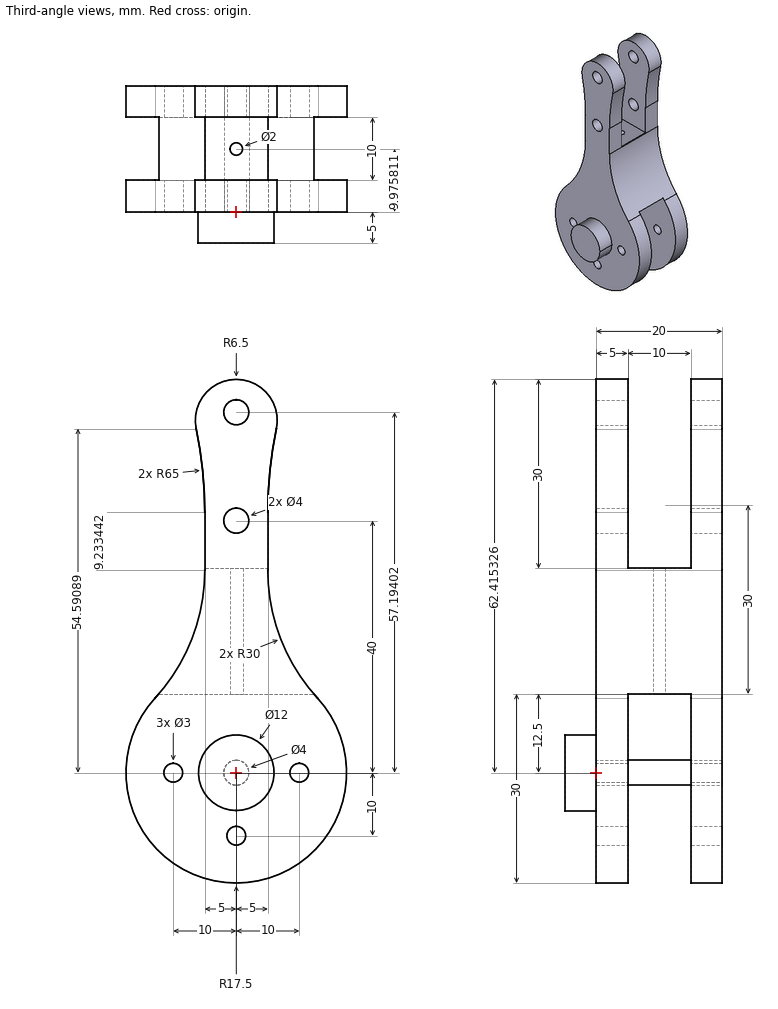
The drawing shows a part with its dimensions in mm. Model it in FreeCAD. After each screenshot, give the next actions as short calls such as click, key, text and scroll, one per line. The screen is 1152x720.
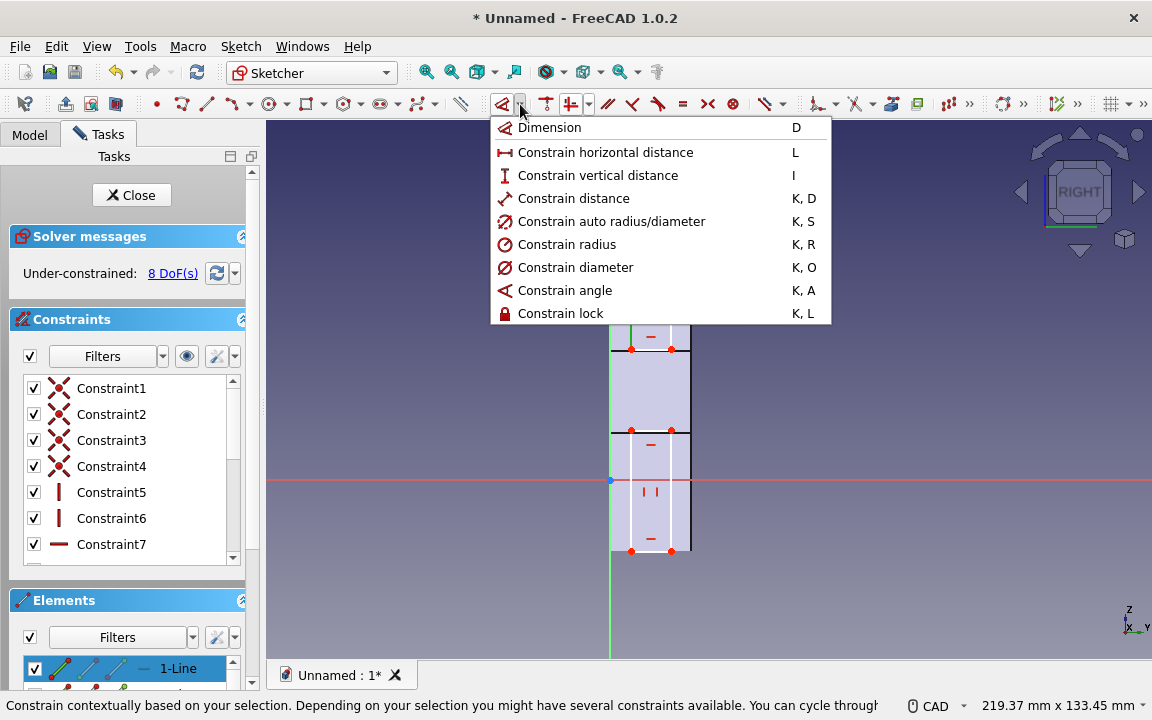
click(661, 176)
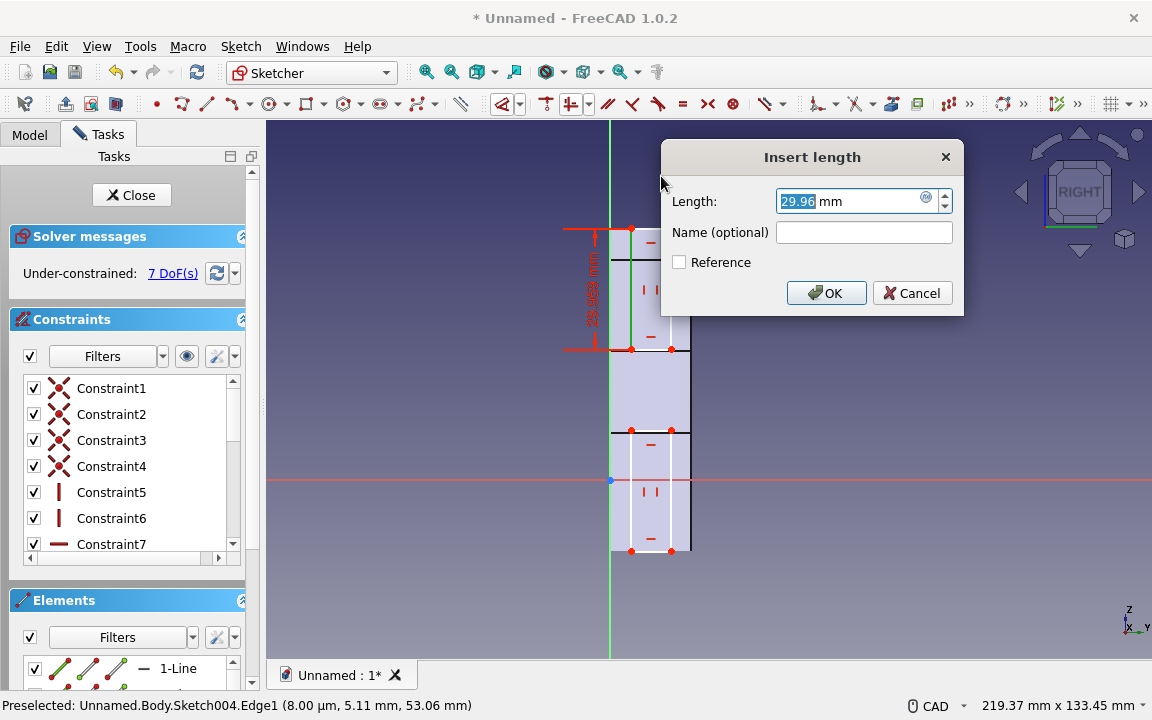
text(30)
key(Return)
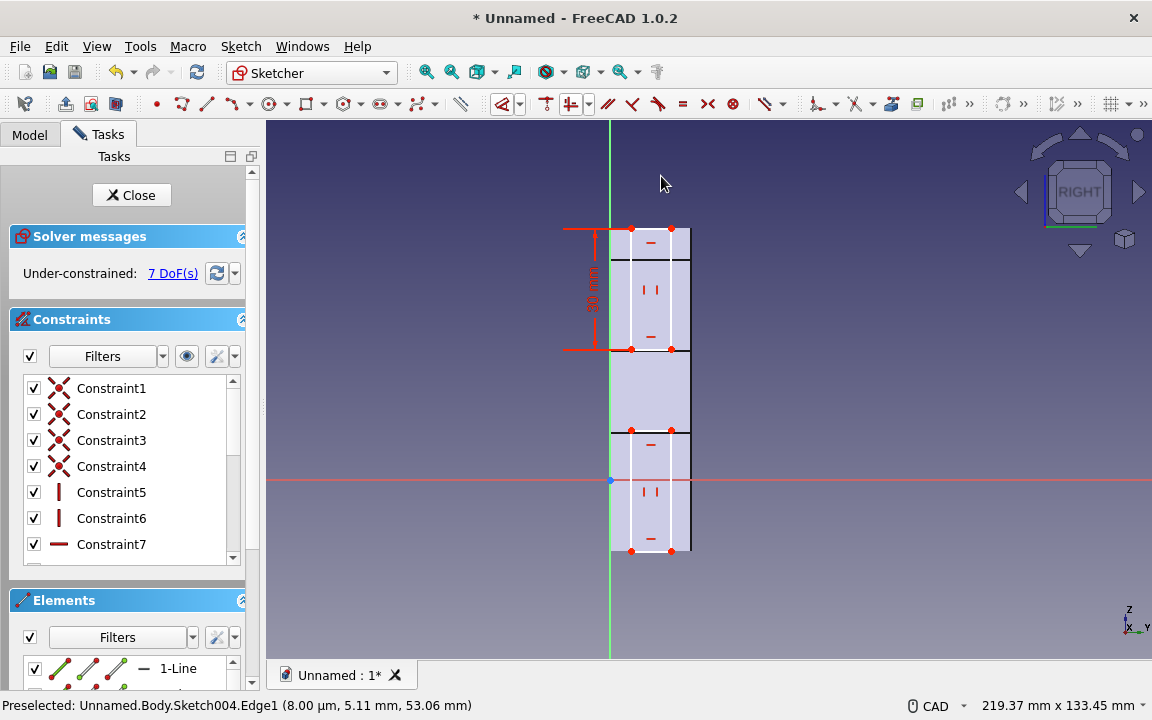
click(643, 350)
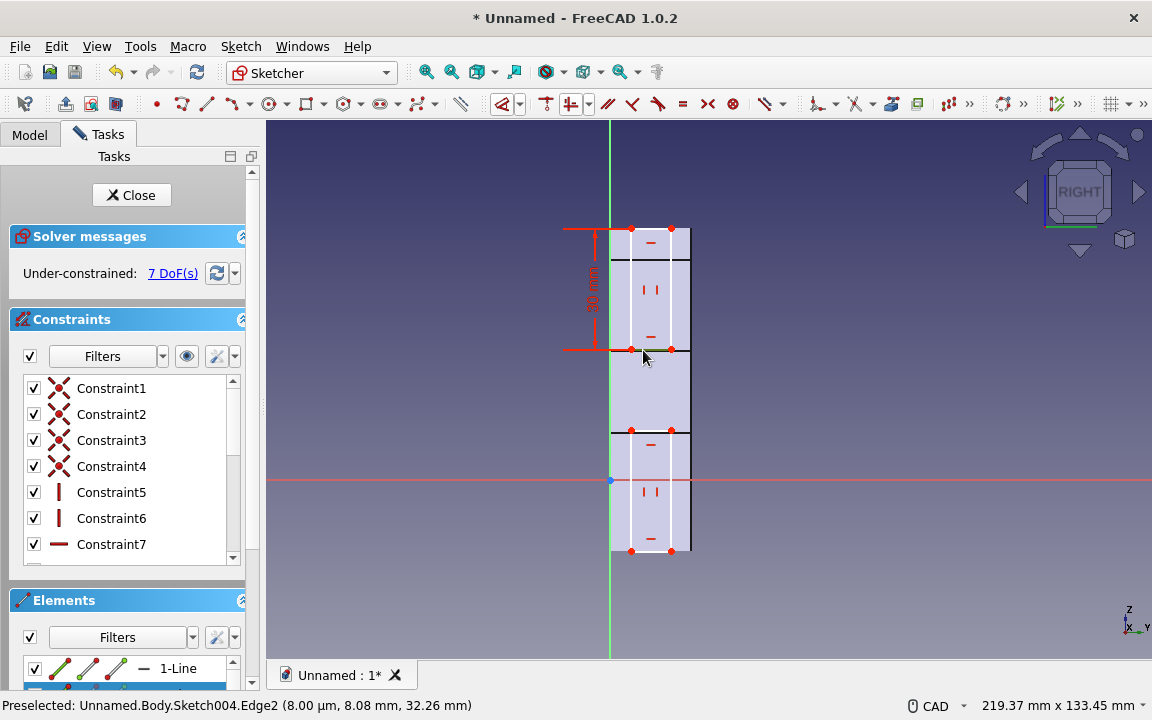
key(l)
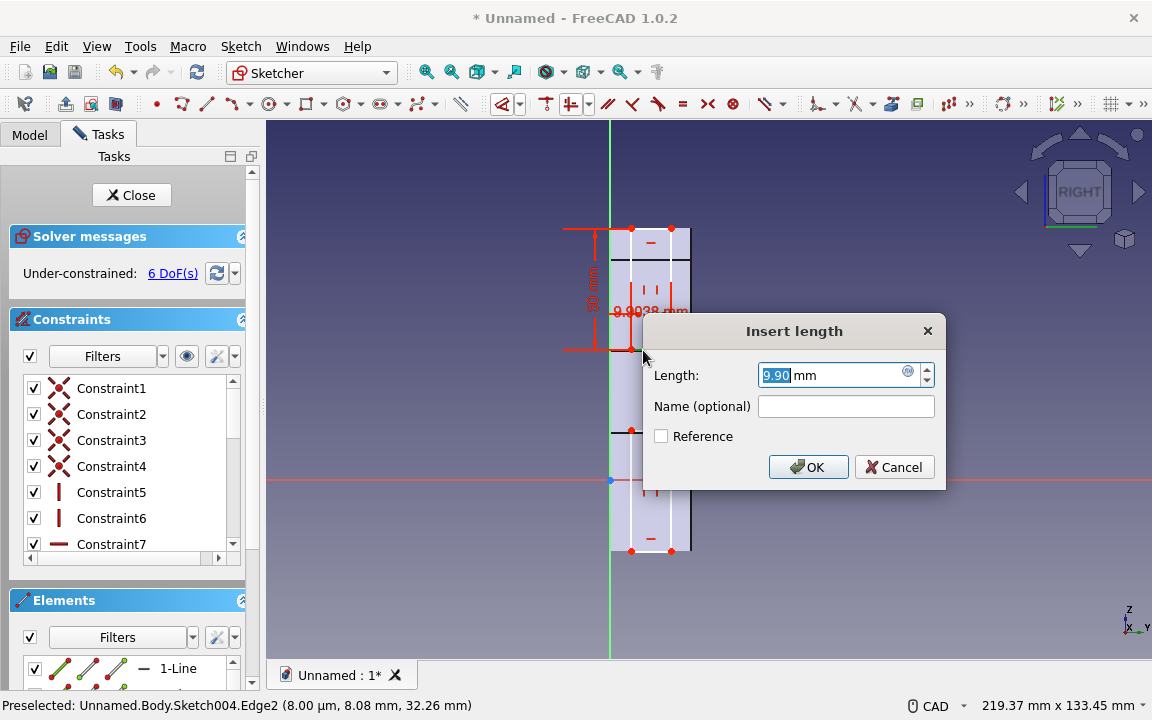
text(10)
key(Return)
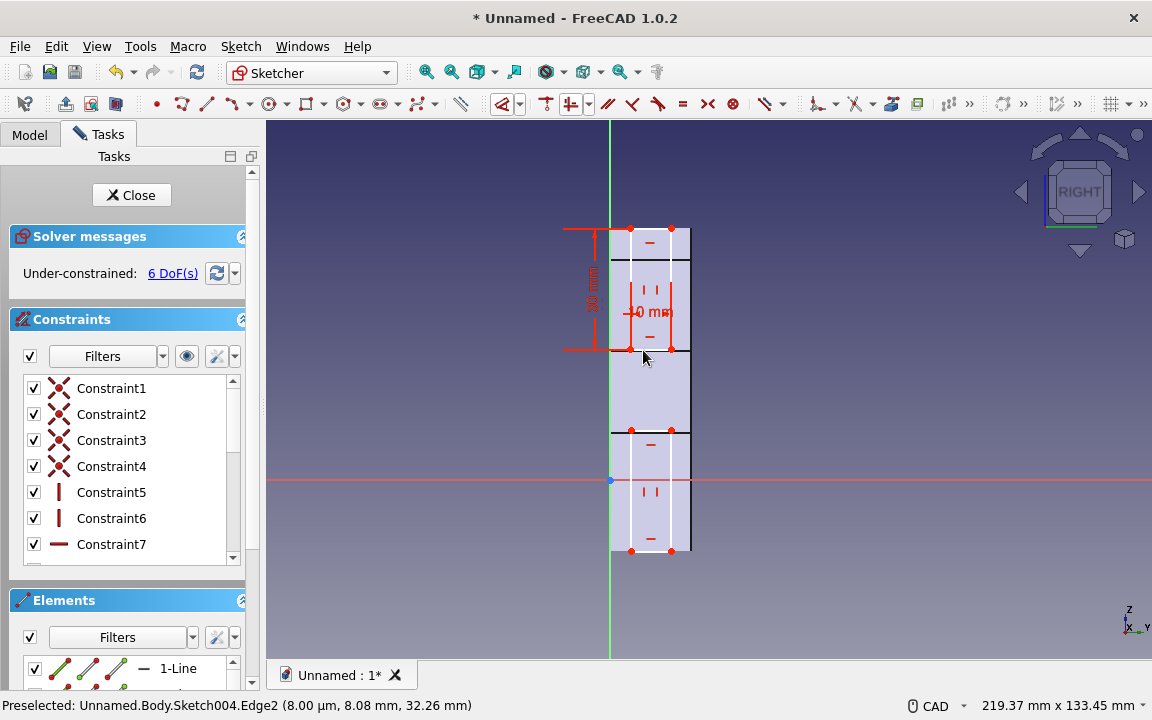
click(631, 467)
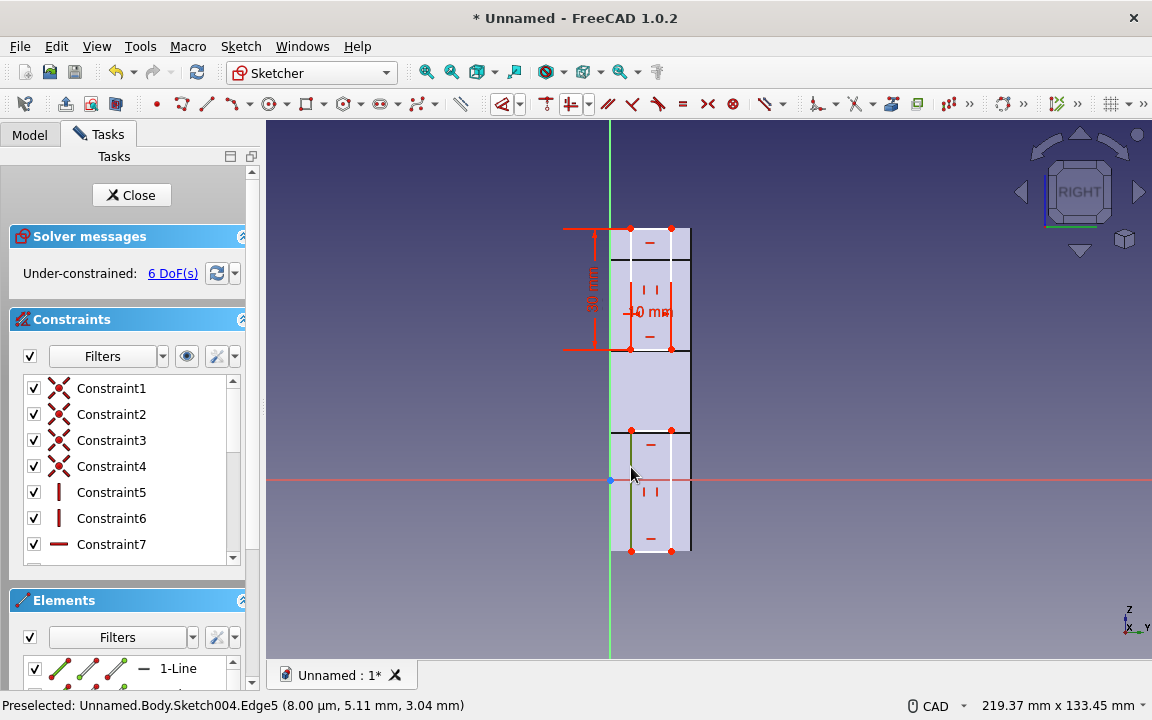
click(520, 104)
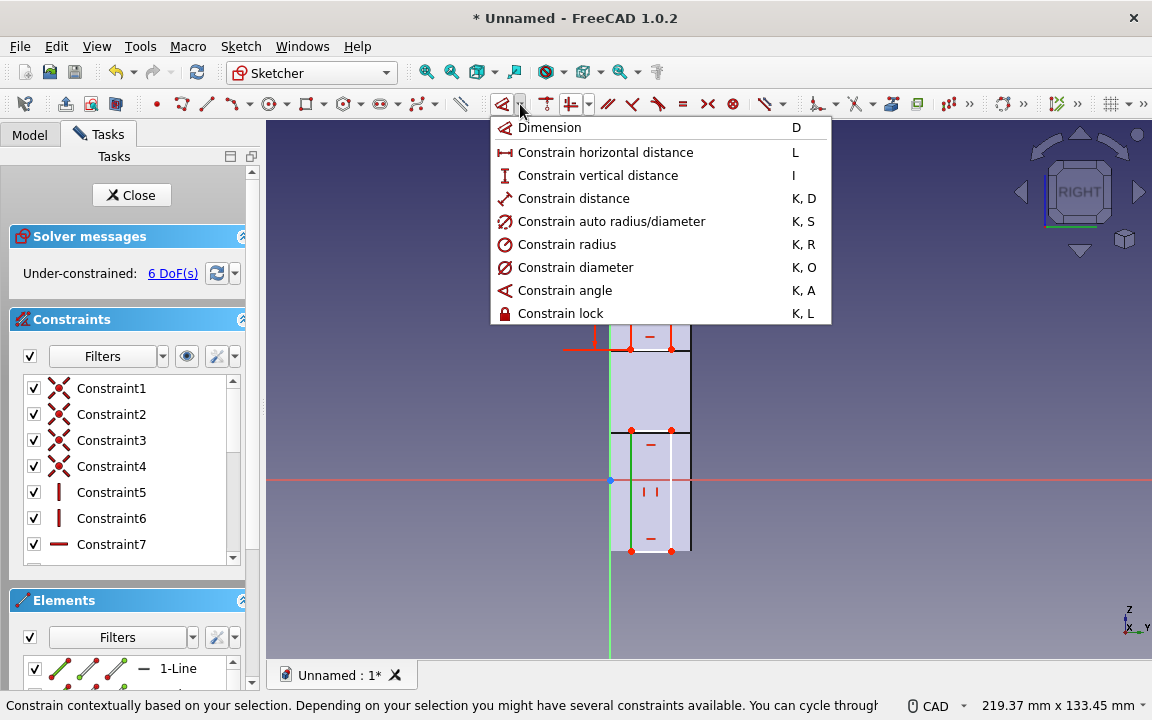
click(661, 176)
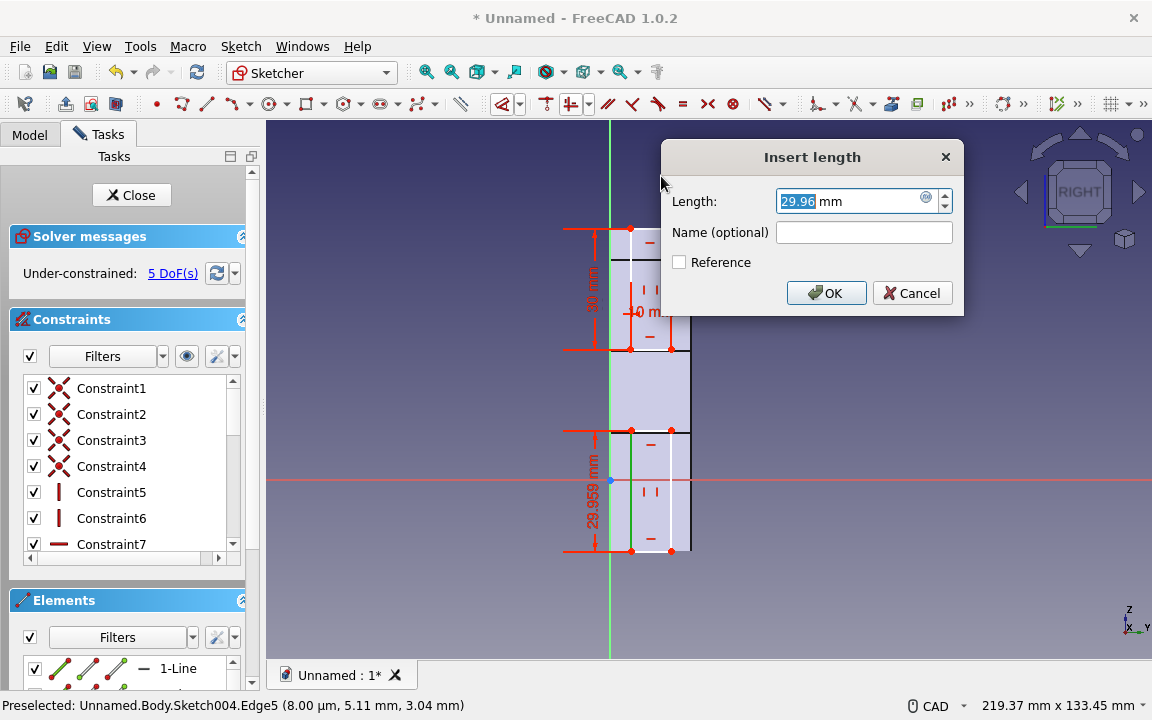
text(30)
key(Return)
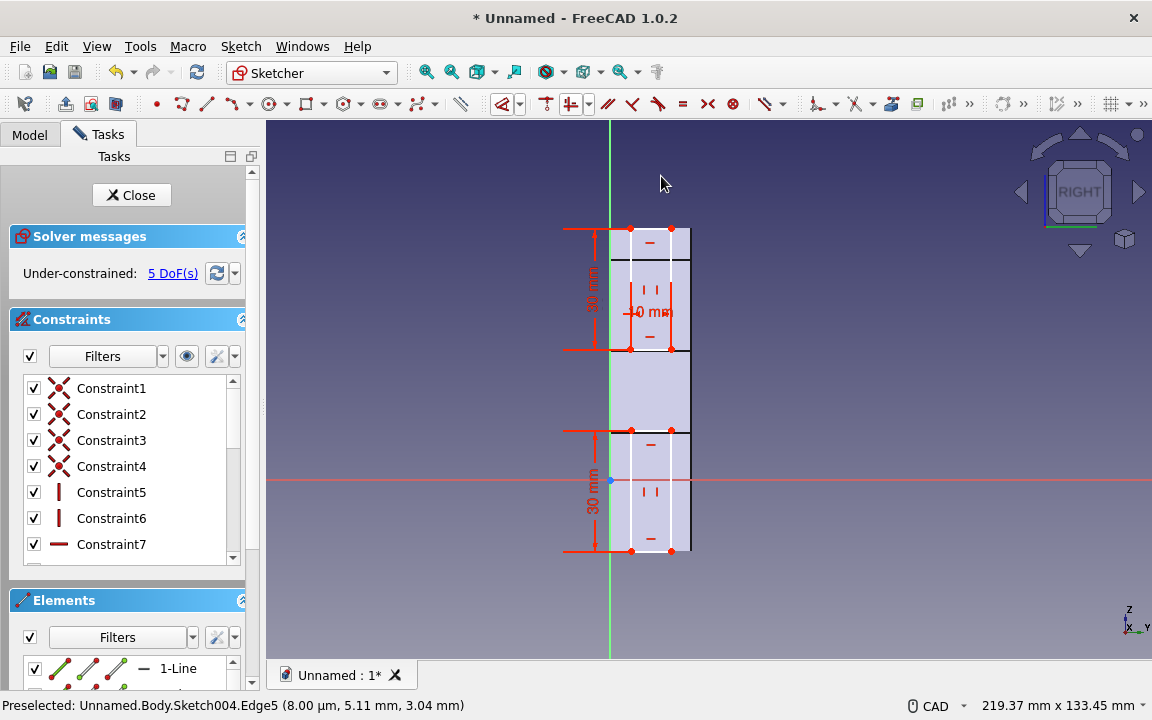
click(643, 552)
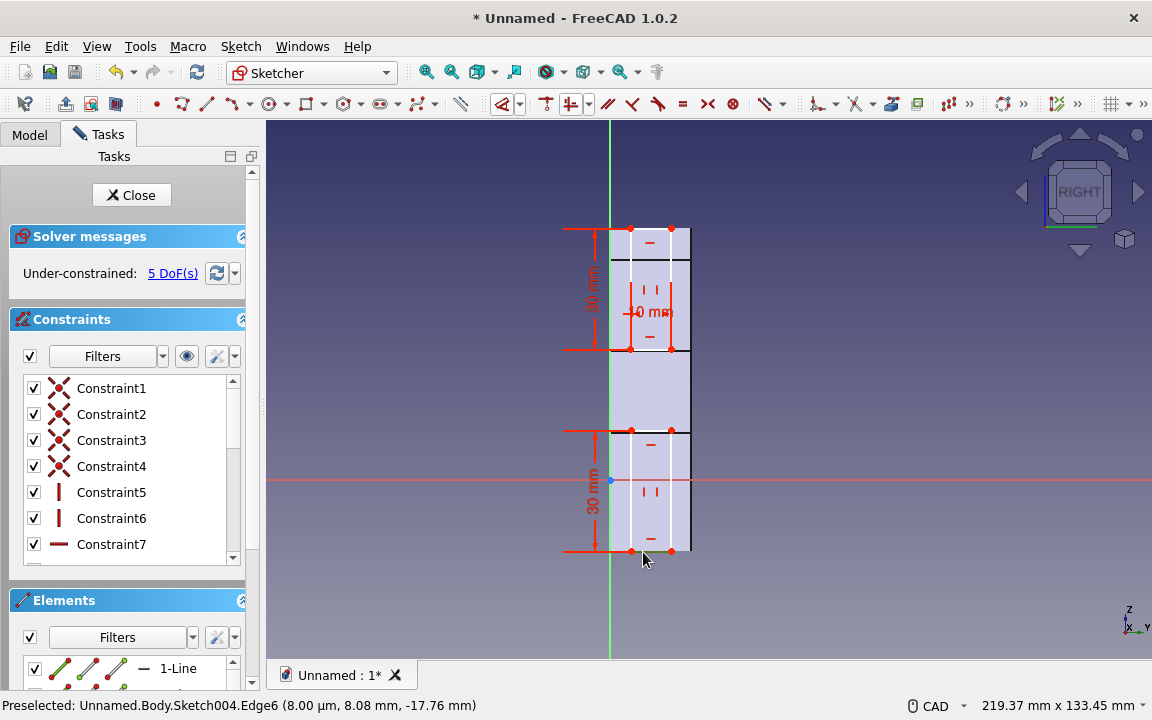
click(520, 104)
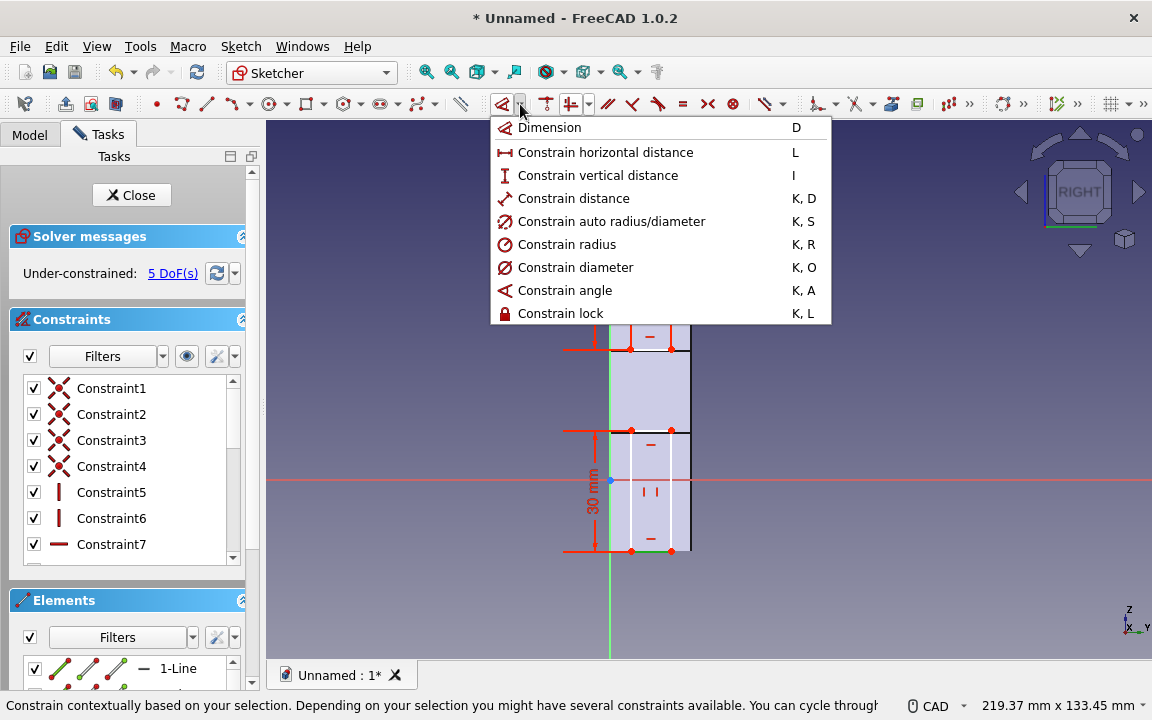
click(661, 152)